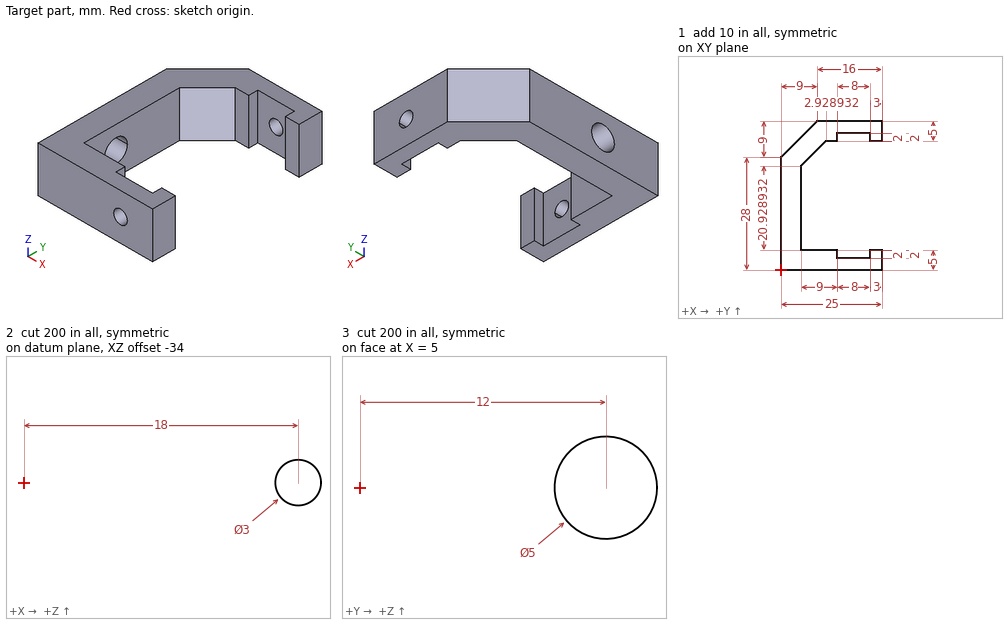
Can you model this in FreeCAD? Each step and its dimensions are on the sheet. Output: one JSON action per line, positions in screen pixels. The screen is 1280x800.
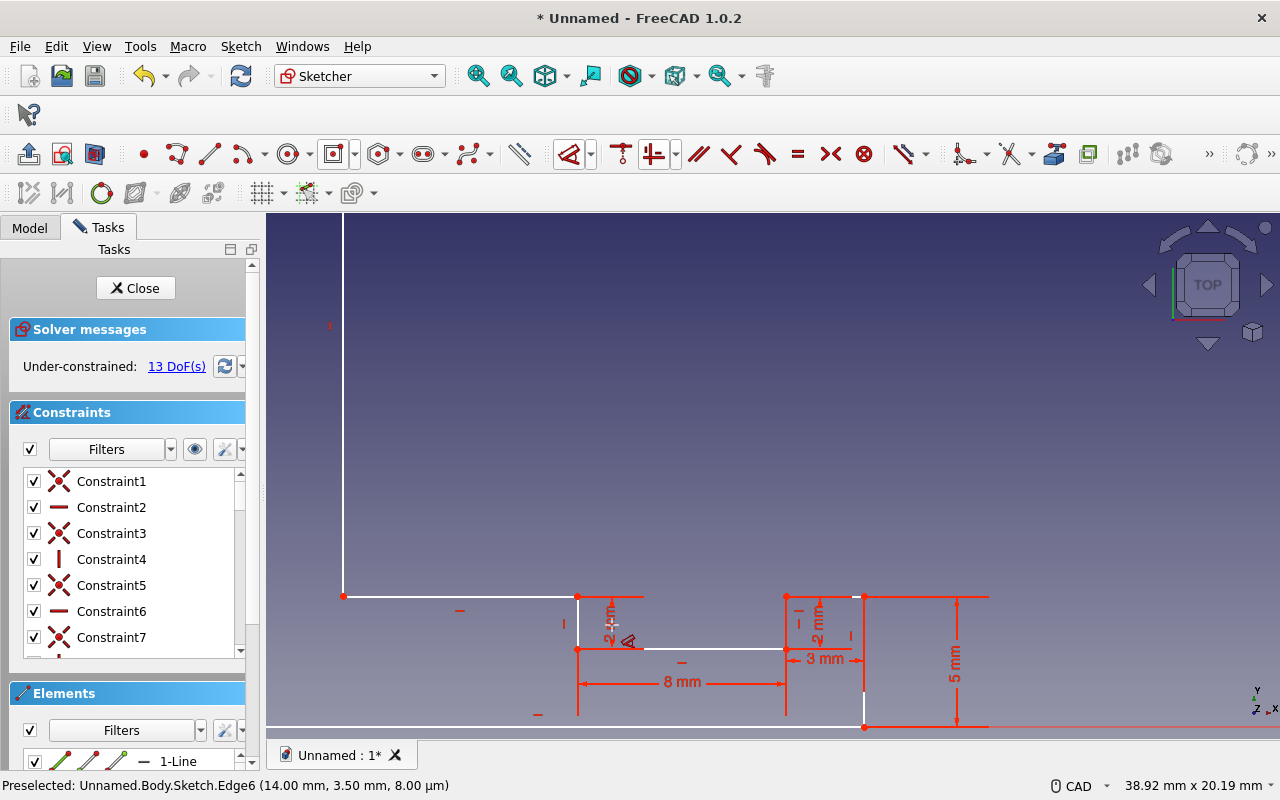
{"action": "left_click", "coordinate": [507, 597]}
{"action": "left_click", "coordinate": [461, 631]}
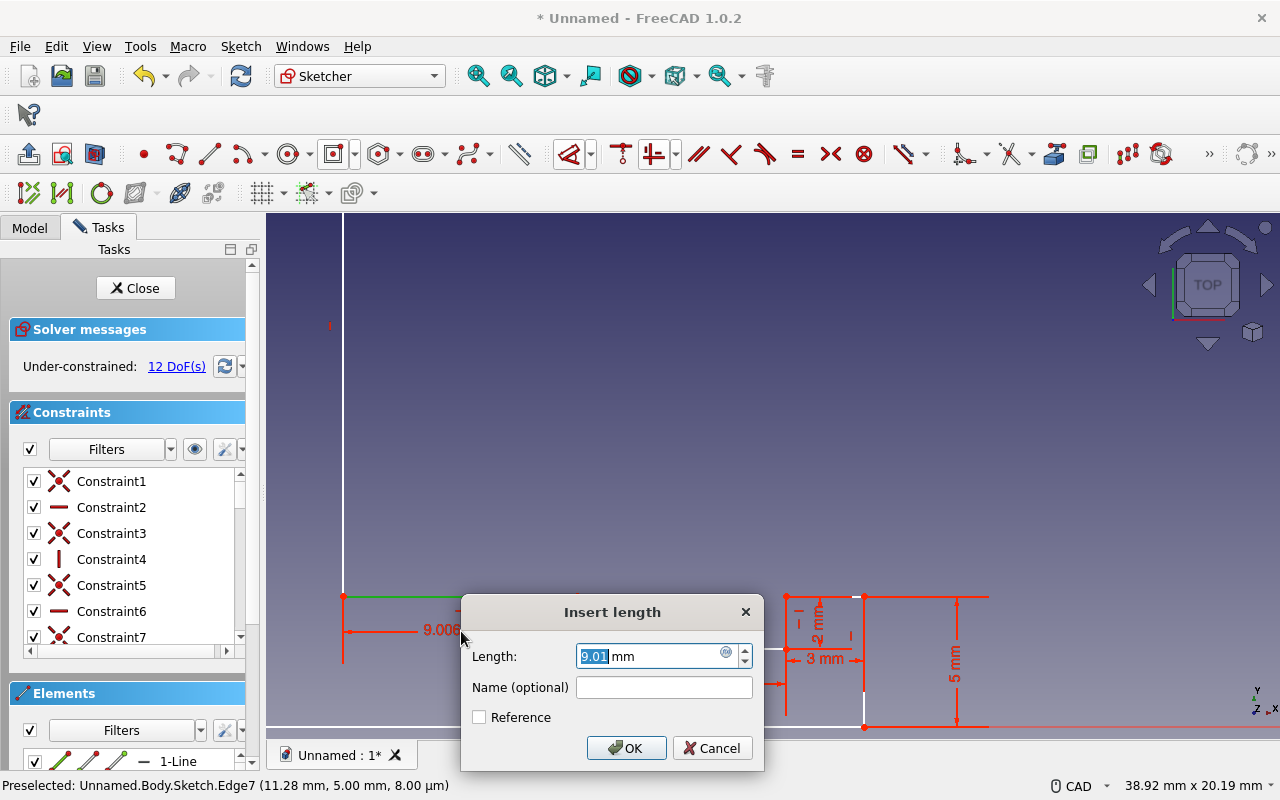
{"action": "type", "text": "9"}
{"action": "key", "text": "Return"}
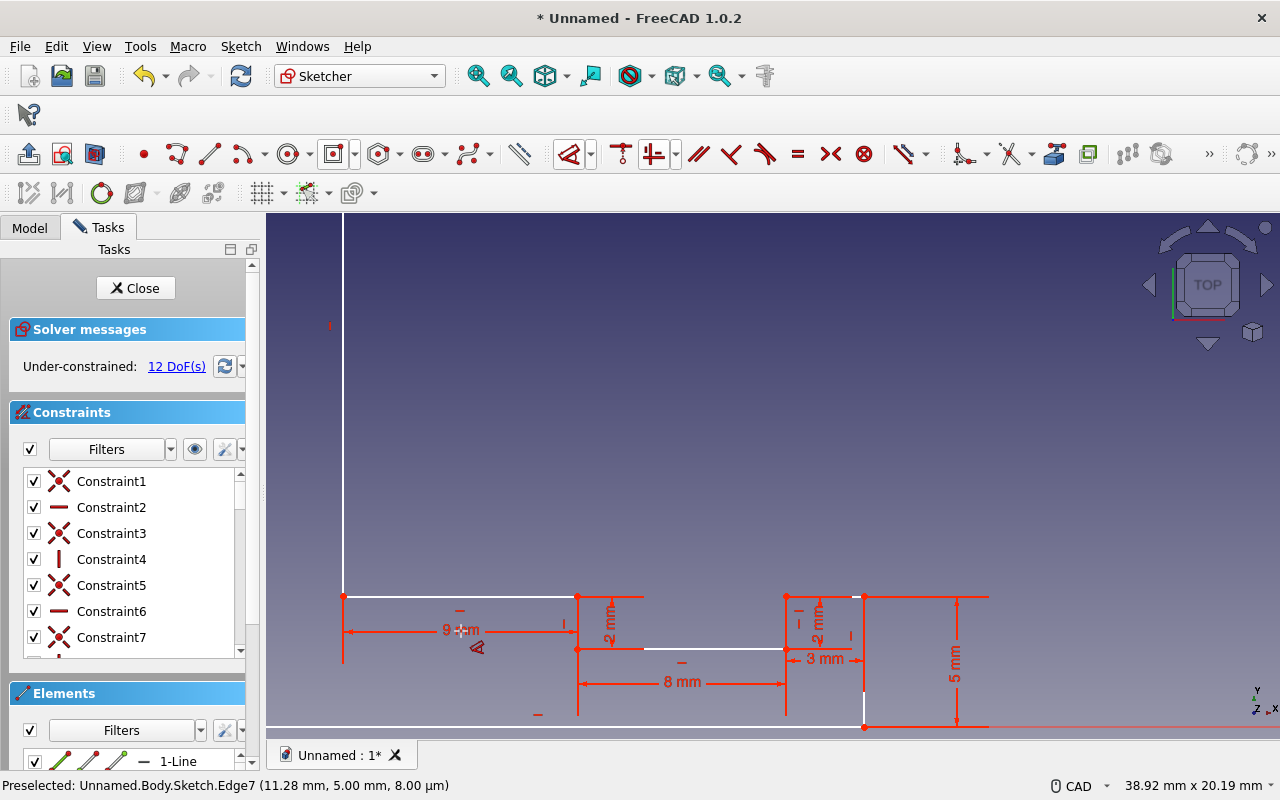
{"action": "scroll", "coordinate": [801, 610], "scroll_direction": "down", "scroll_amount": 5}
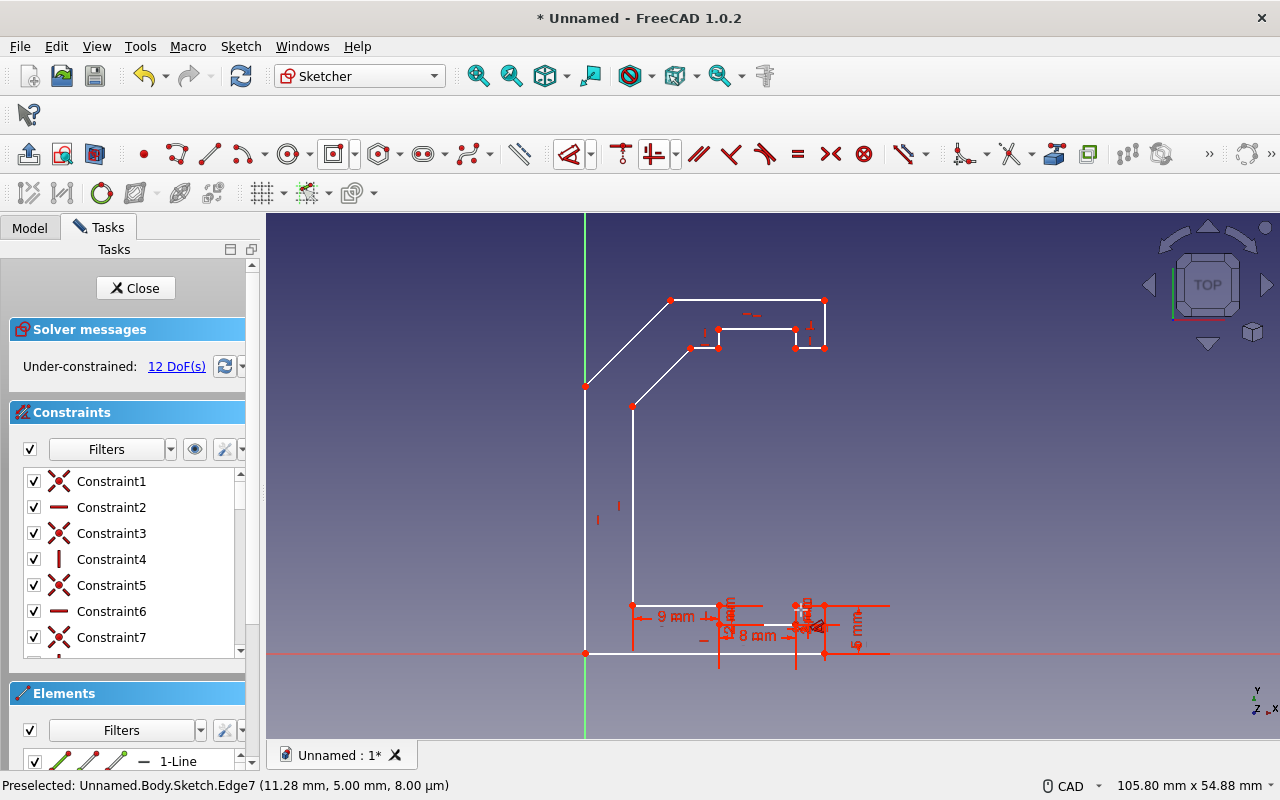
{"action": "scroll", "coordinate": [719, 342], "scroll_direction": "up", "scroll_amount": 5}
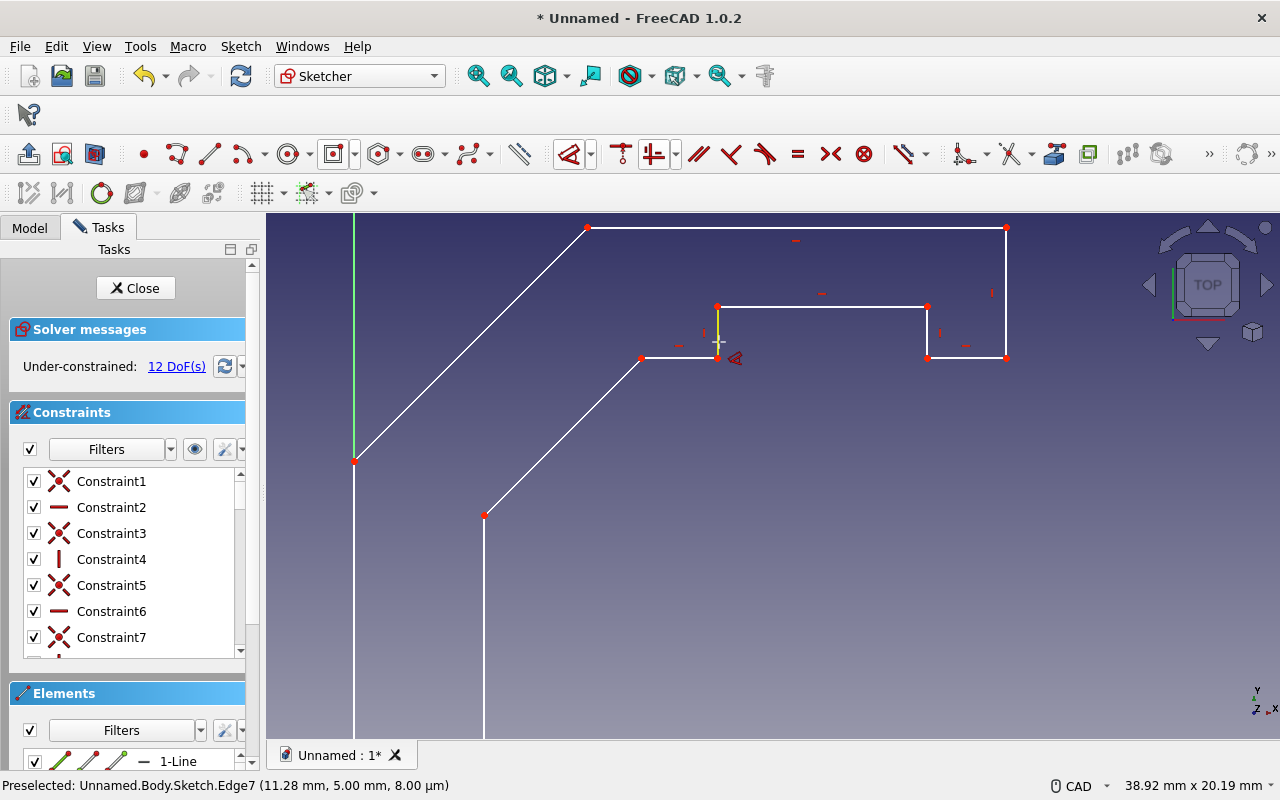
{"action": "left_click", "coordinate": [718, 343]}
{"action": "left_click", "coordinate": [752, 332]}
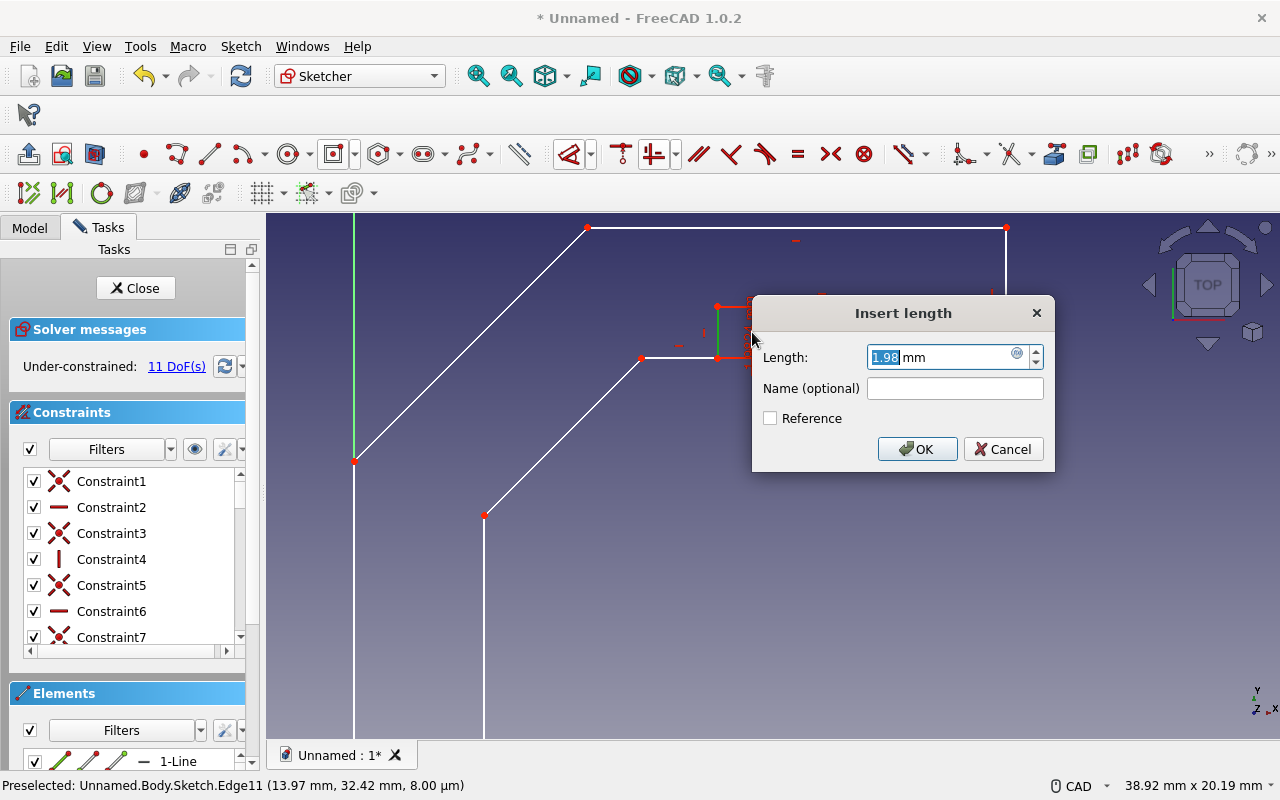
{"action": "type", "text": "2"}
{"action": "key", "text": "Return"}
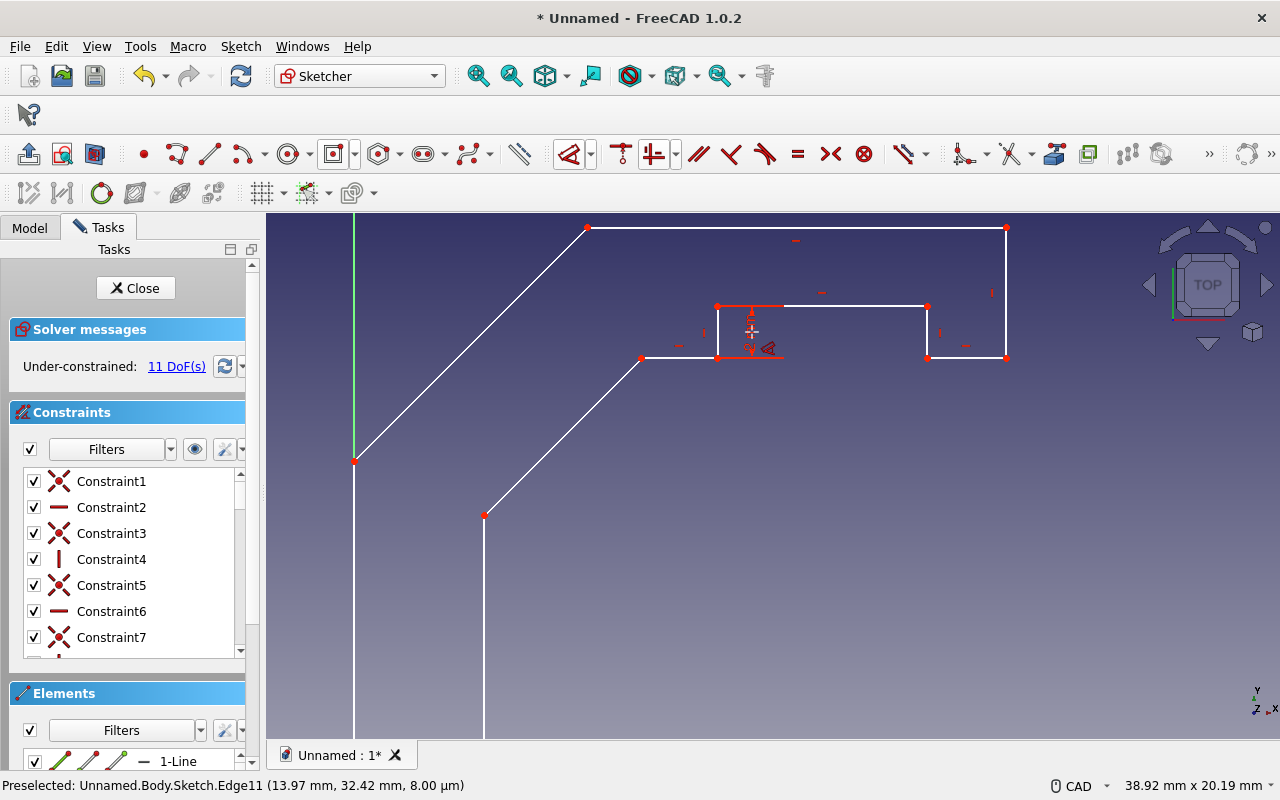
{"action": "left_click", "coordinate": [781, 306]}
{"action": "left_click", "coordinate": [823, 272]}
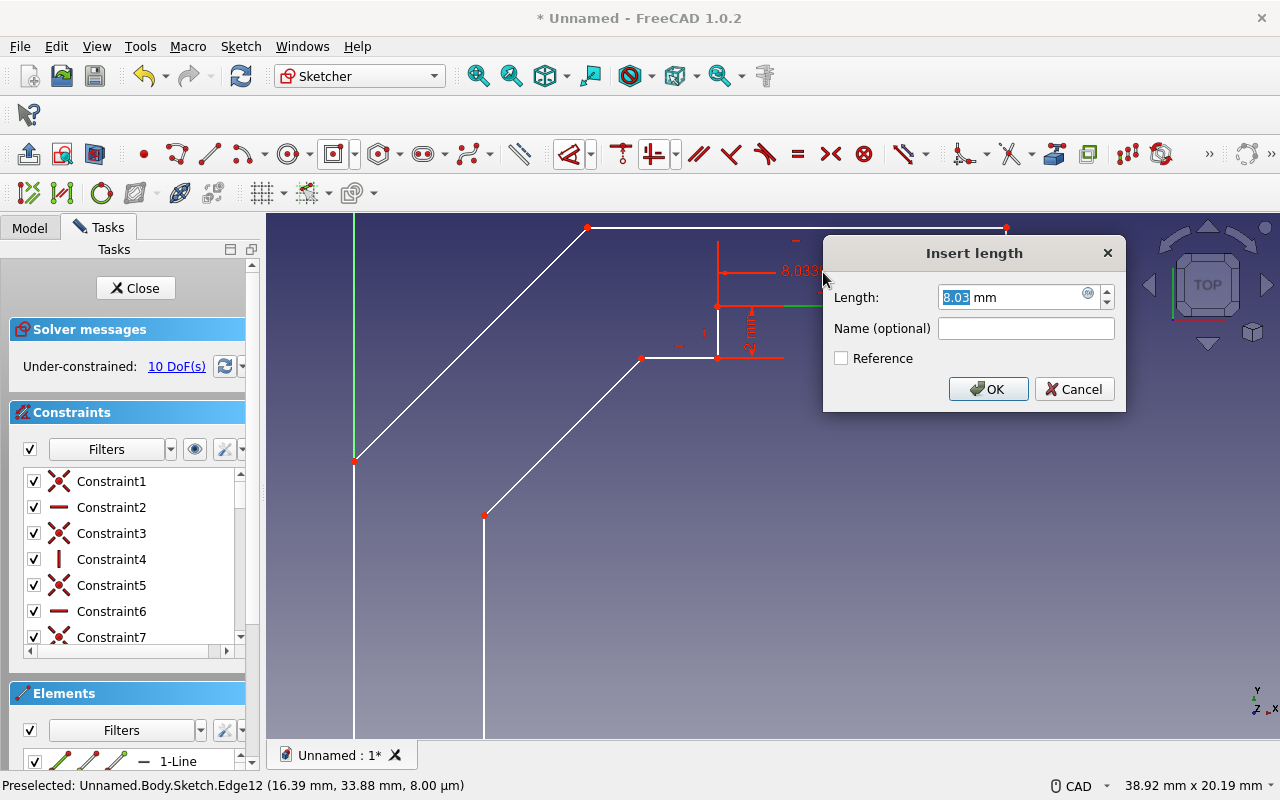
{"action": "type", "text": "8"}
{"action": "key", "text": "Return"}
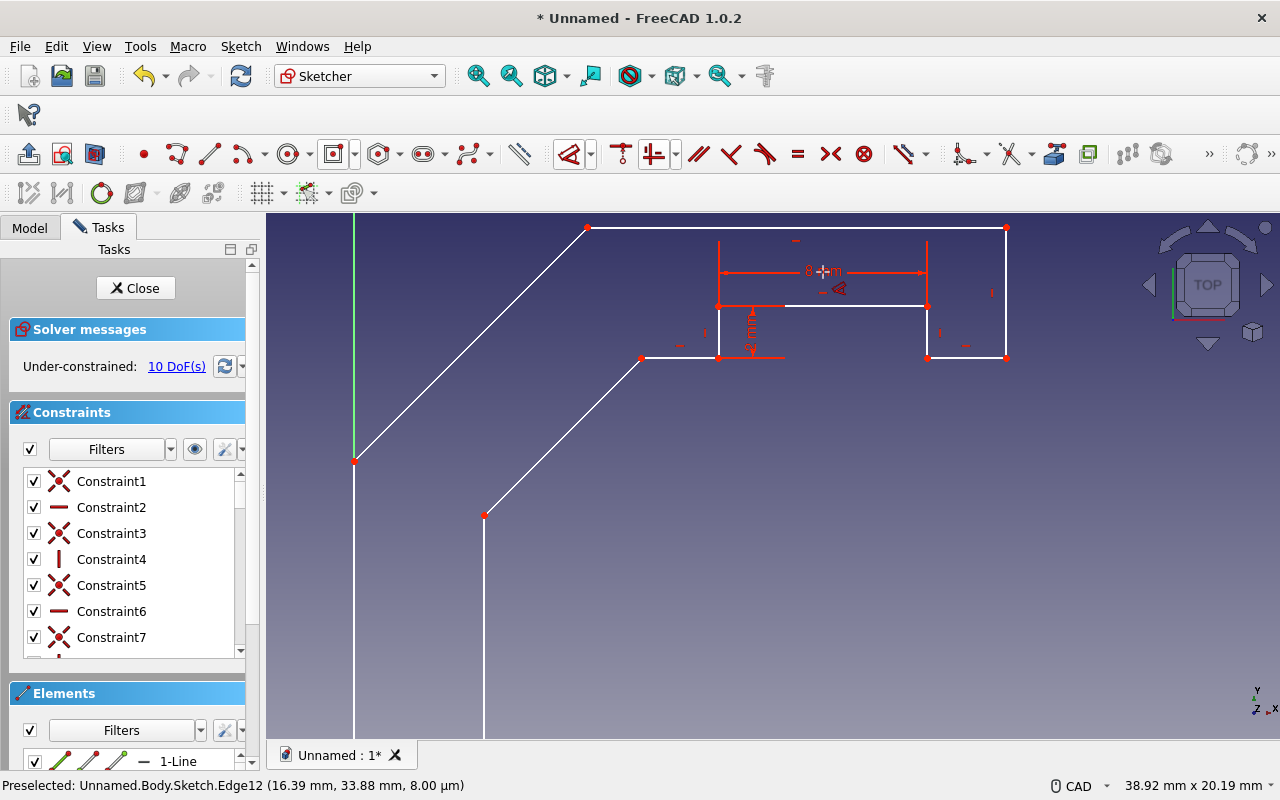
{"action": "left_click", "coordinate": [927, 322]}
{"action": "left_click", "coordinate": [961, 332]}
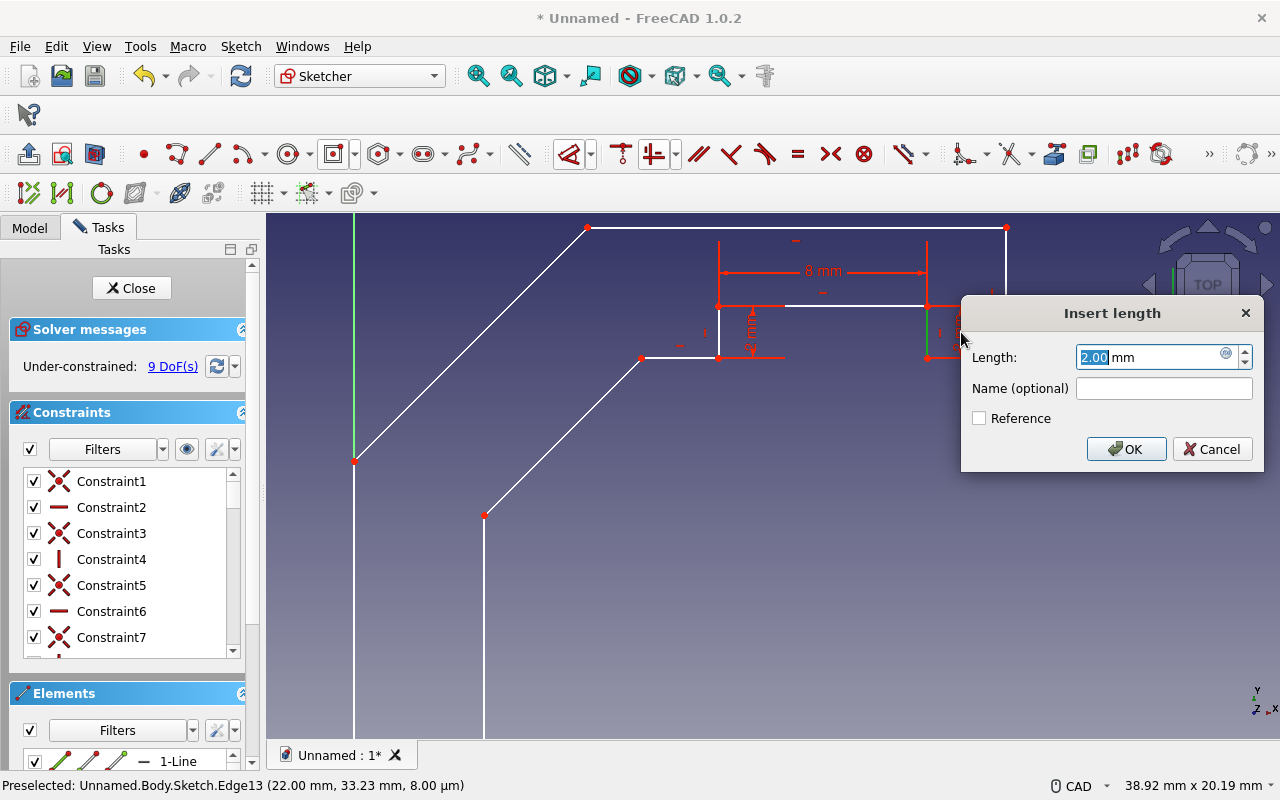
{"action": "type", "text": "2"}
{"action": "key", "text": "Return"}